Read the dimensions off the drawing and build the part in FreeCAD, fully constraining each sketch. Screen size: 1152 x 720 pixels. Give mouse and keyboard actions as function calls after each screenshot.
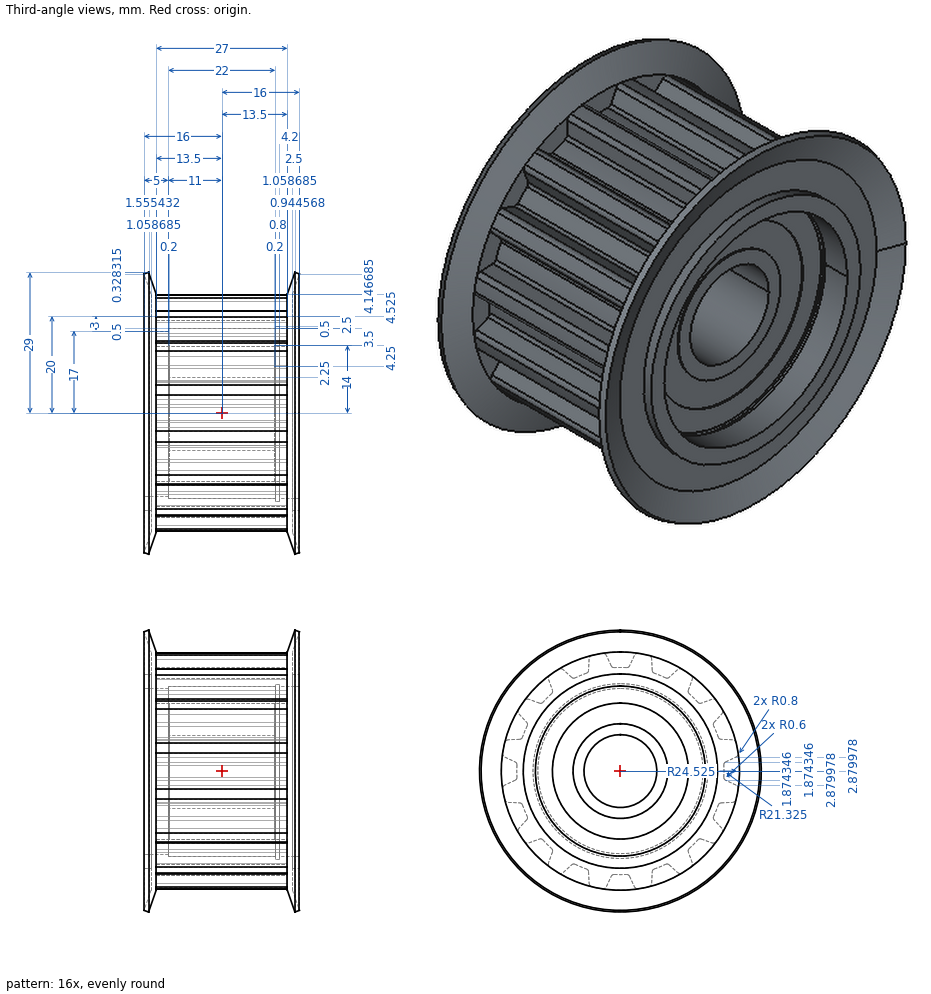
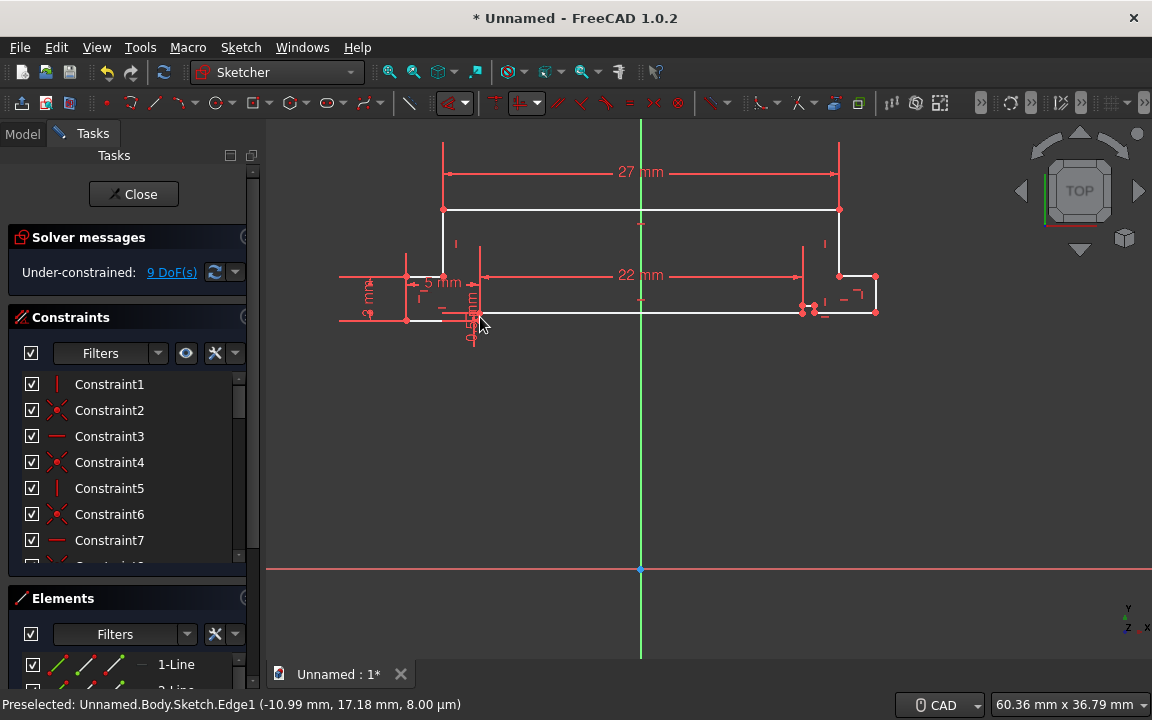
scroll(803, 311, up, 10)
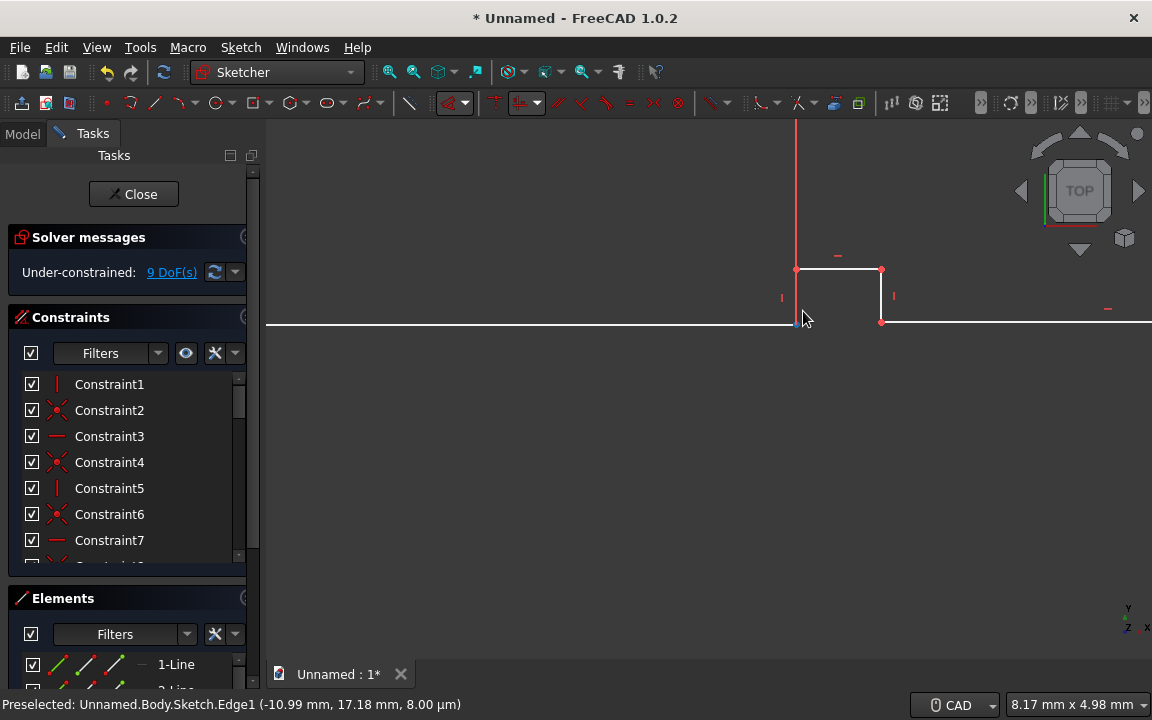
click(796, 308)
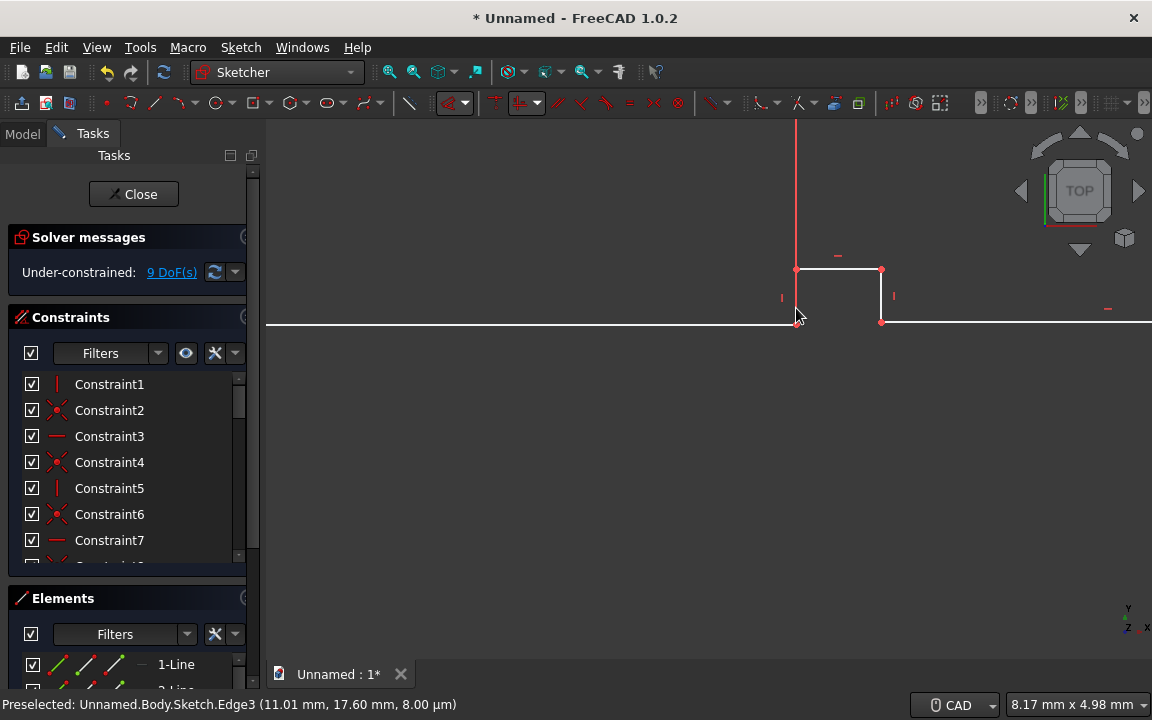
key(i)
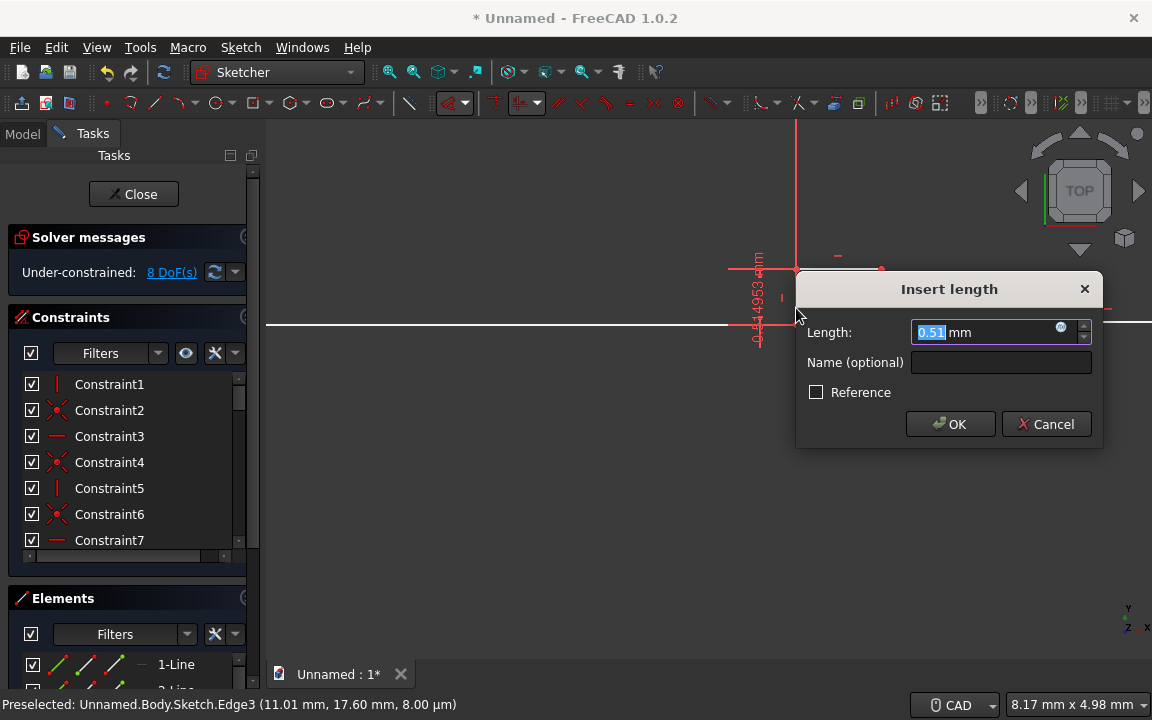
text(0.5)
key(Return)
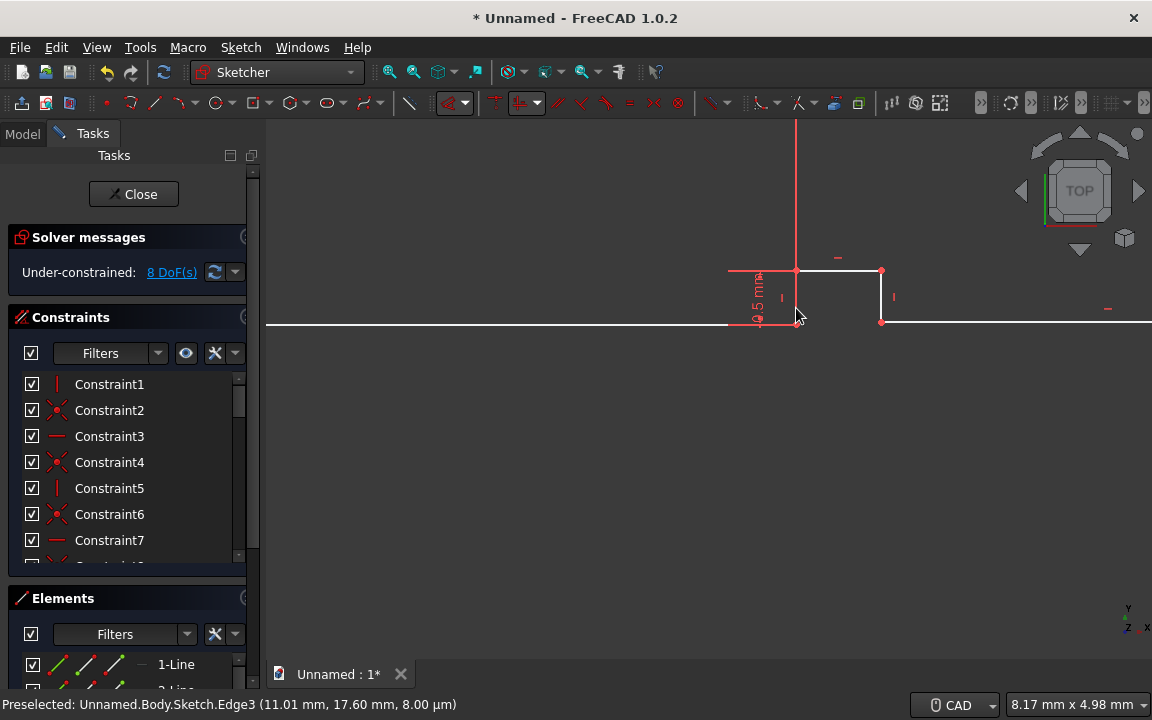
click(822, 271)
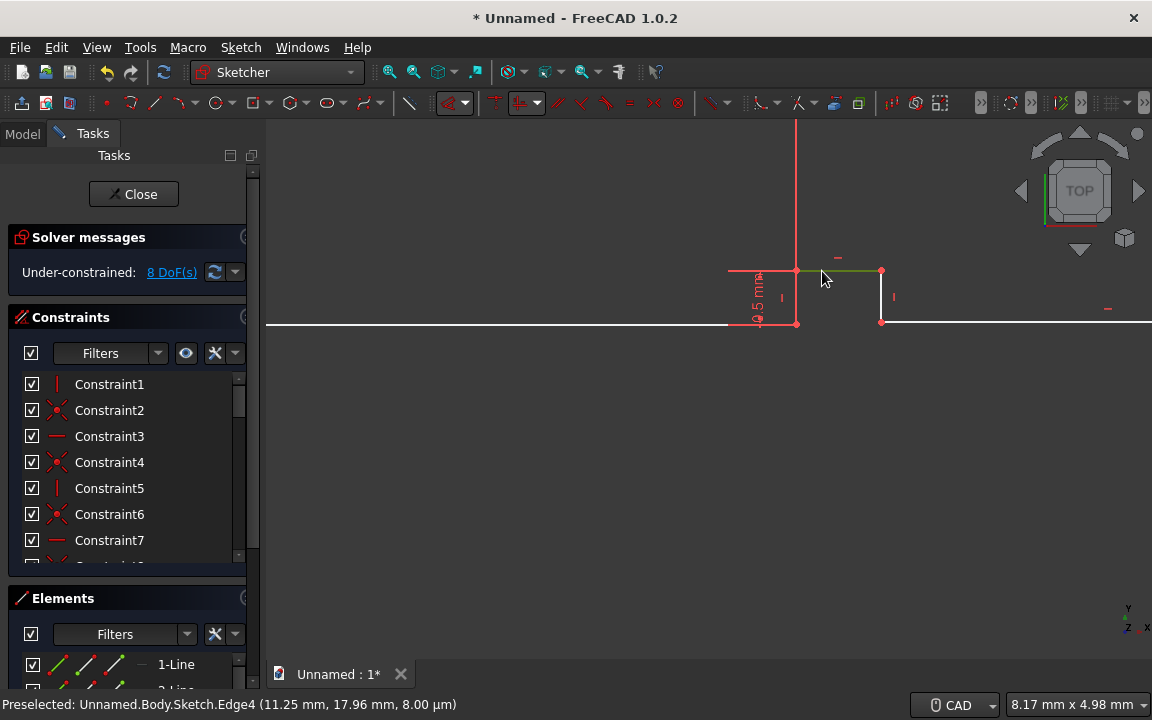
click(468, 104)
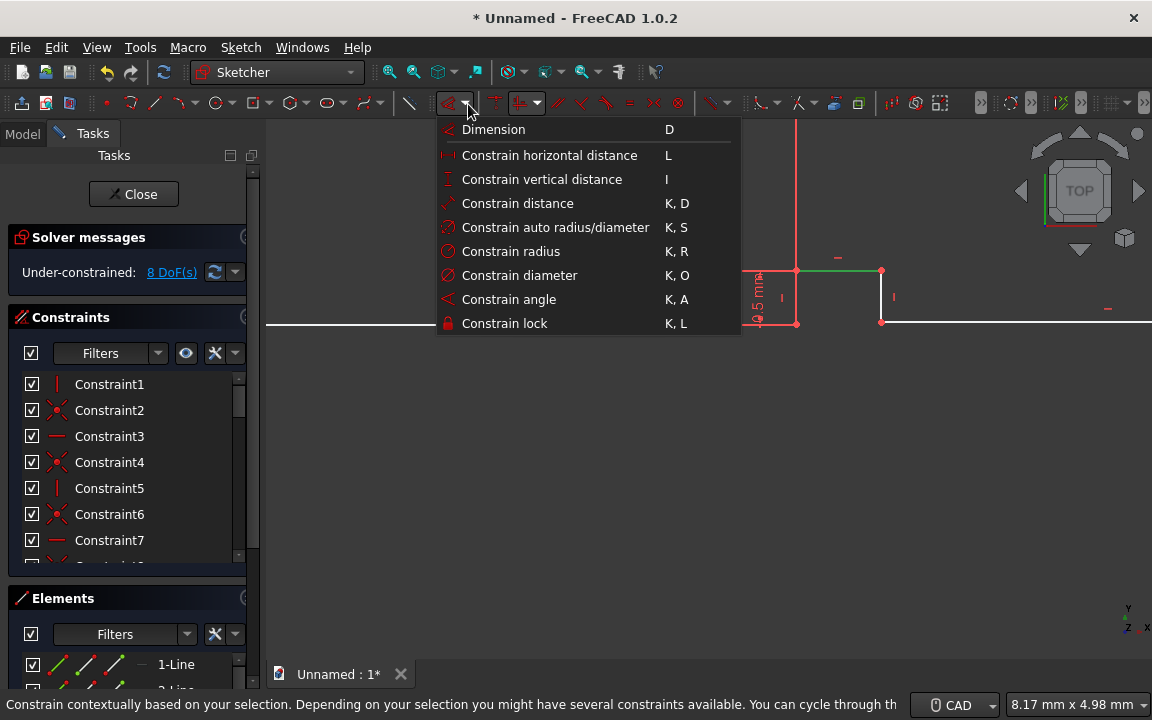
click(589, 155)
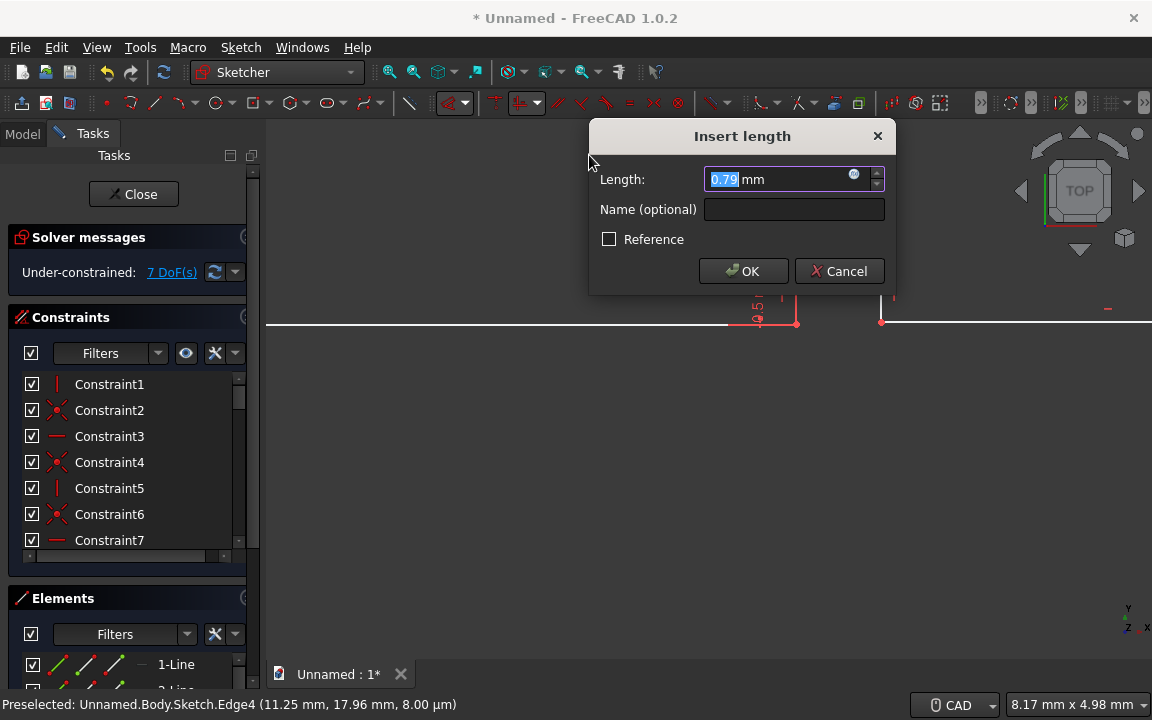
text(0.8)
key(Return)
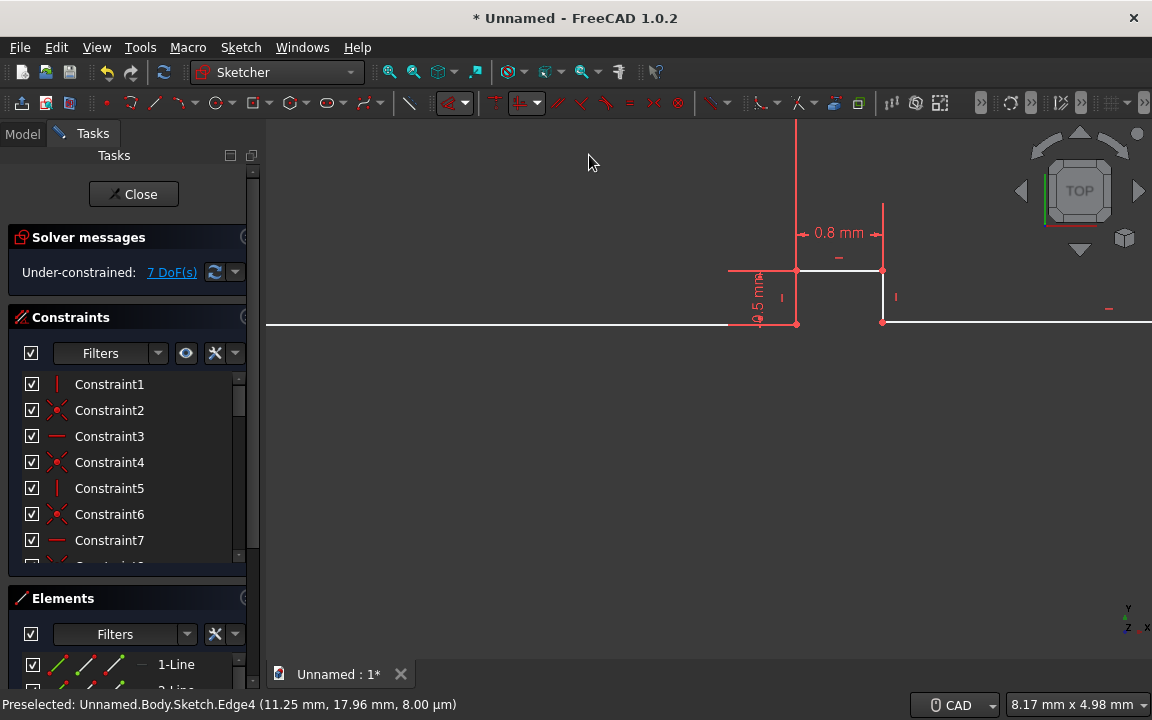
click(883, 286)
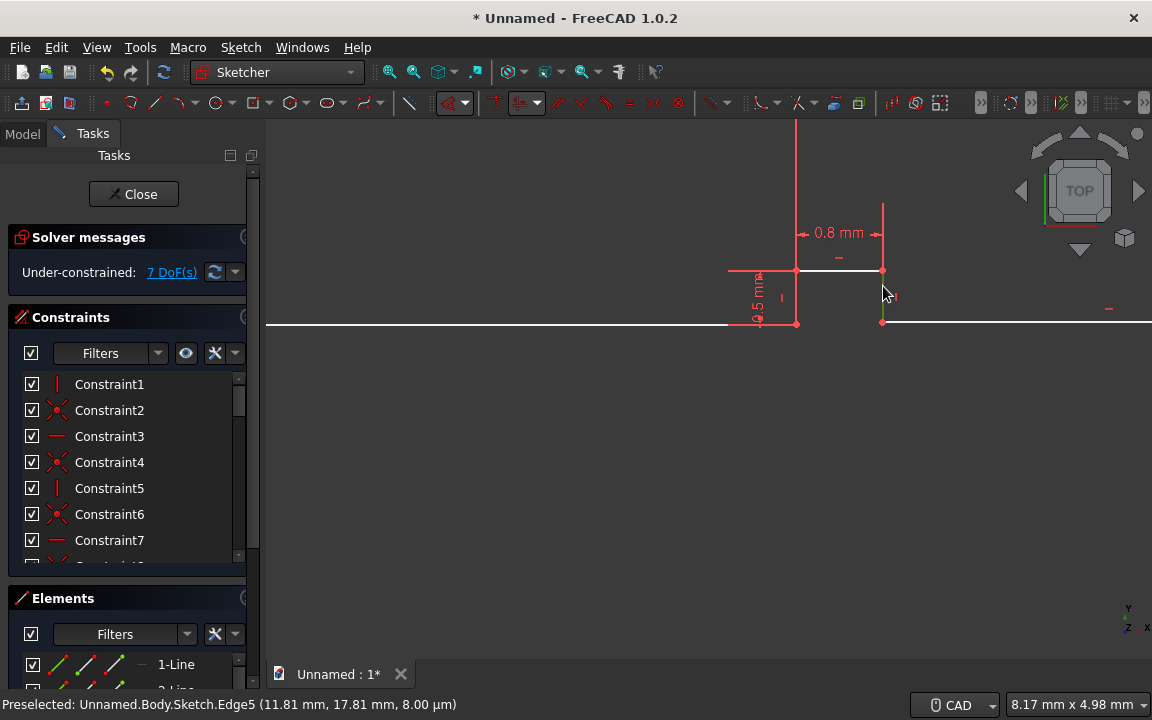
key(i)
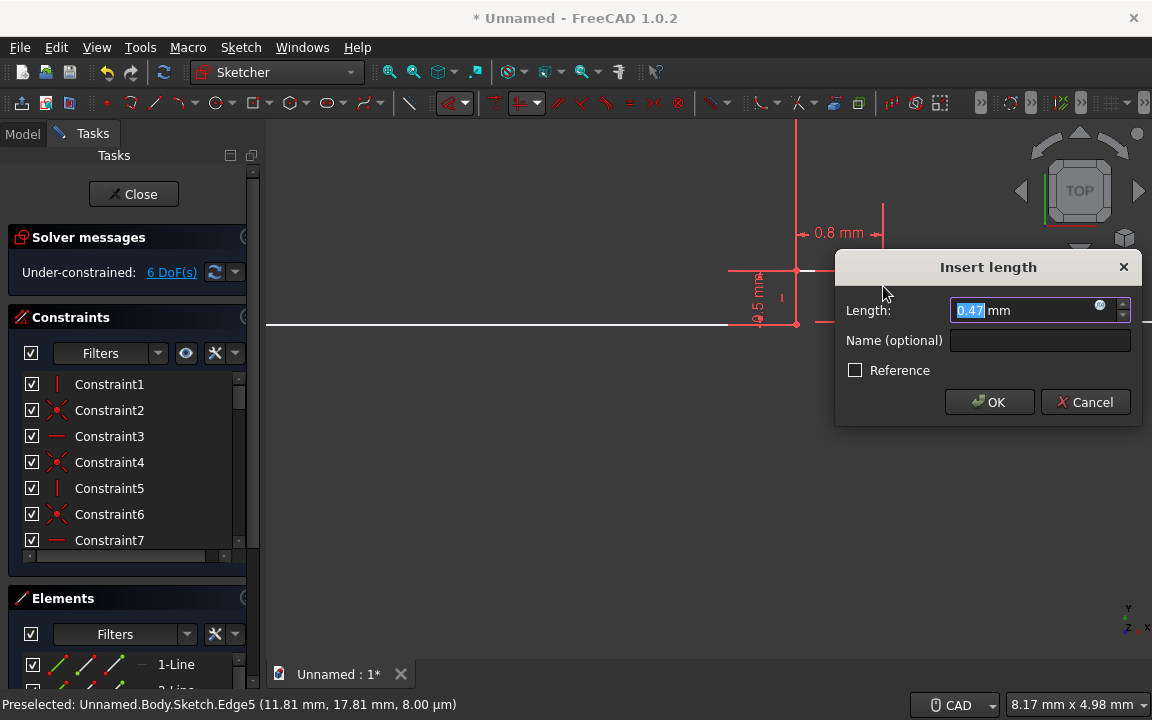
text(0.5)
key(Return)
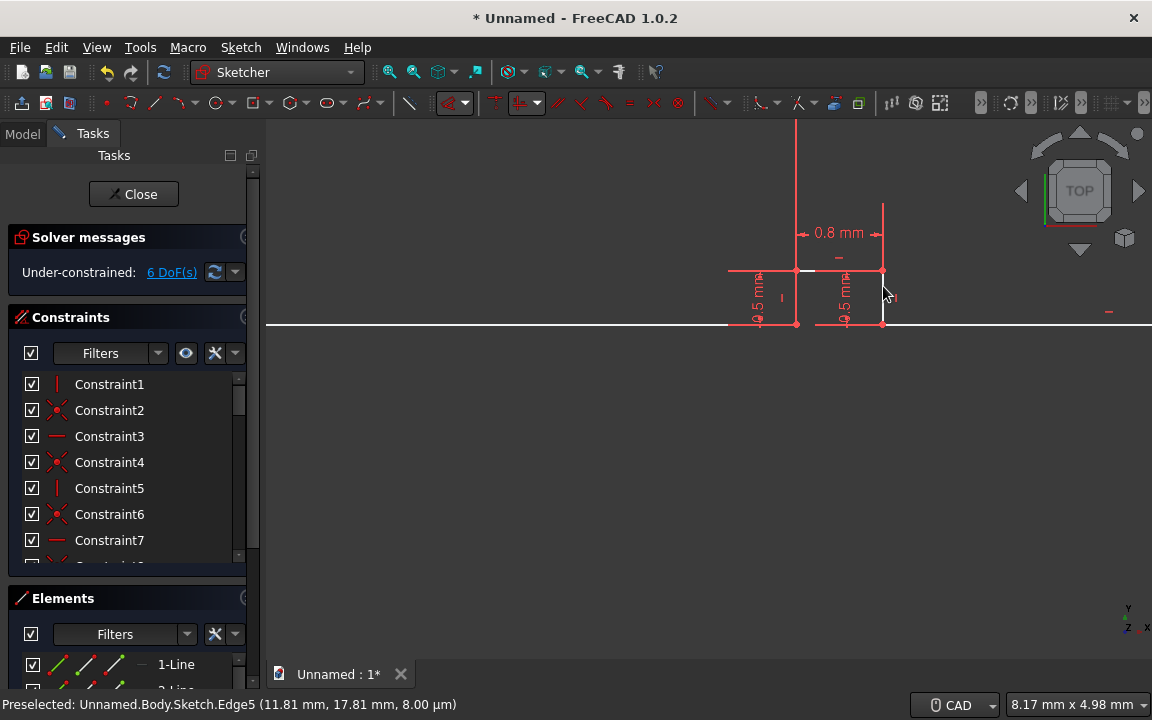
scroll(803, 311, down, 10)